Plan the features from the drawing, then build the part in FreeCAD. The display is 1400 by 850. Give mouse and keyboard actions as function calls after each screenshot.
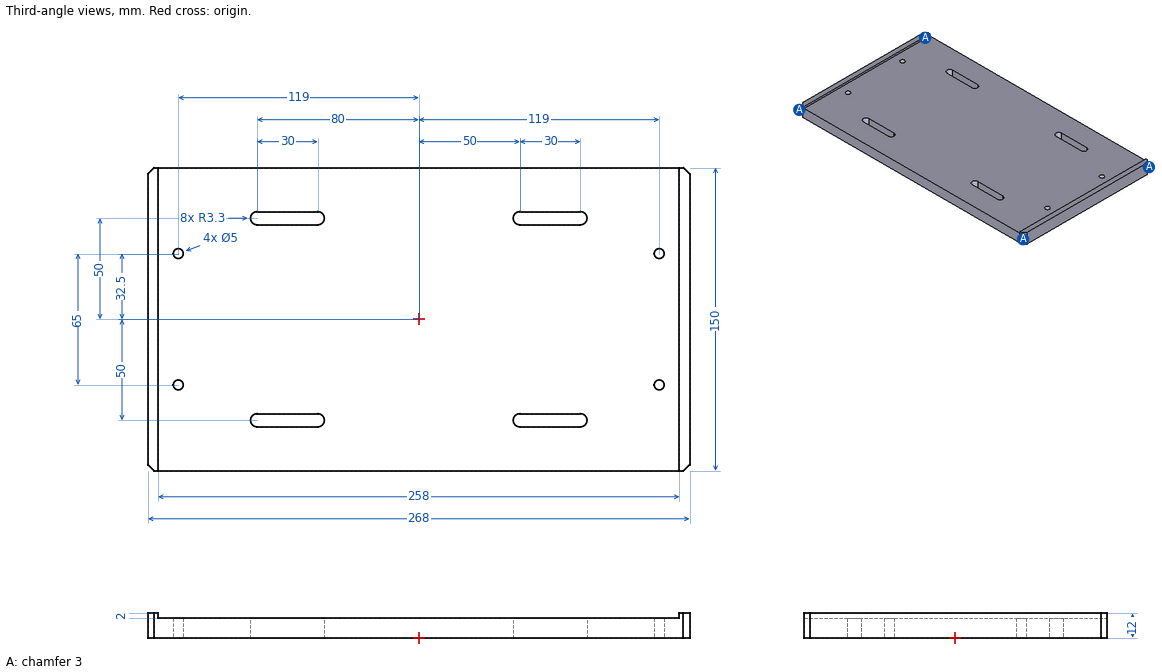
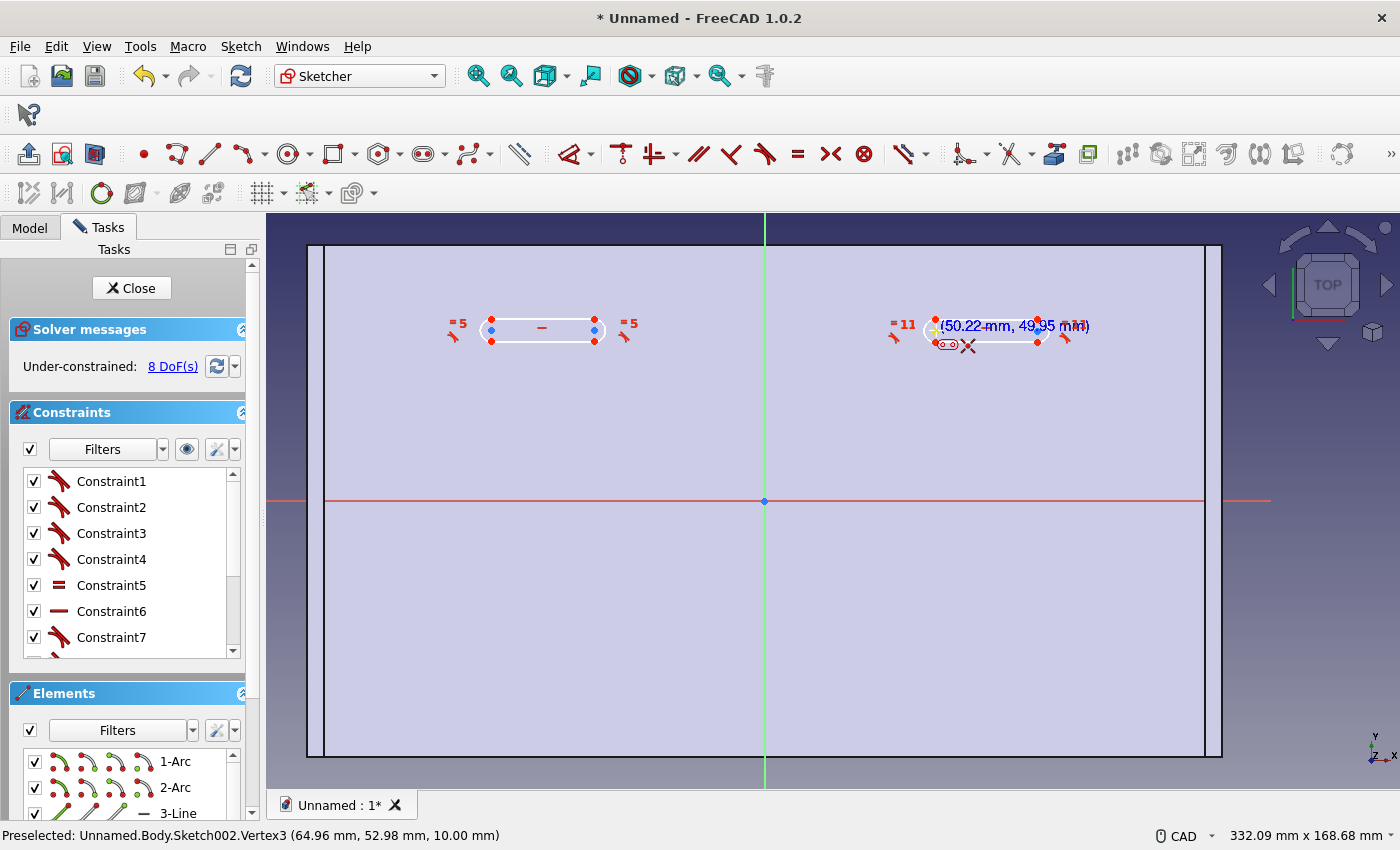
scroll(492, 672, up, 4)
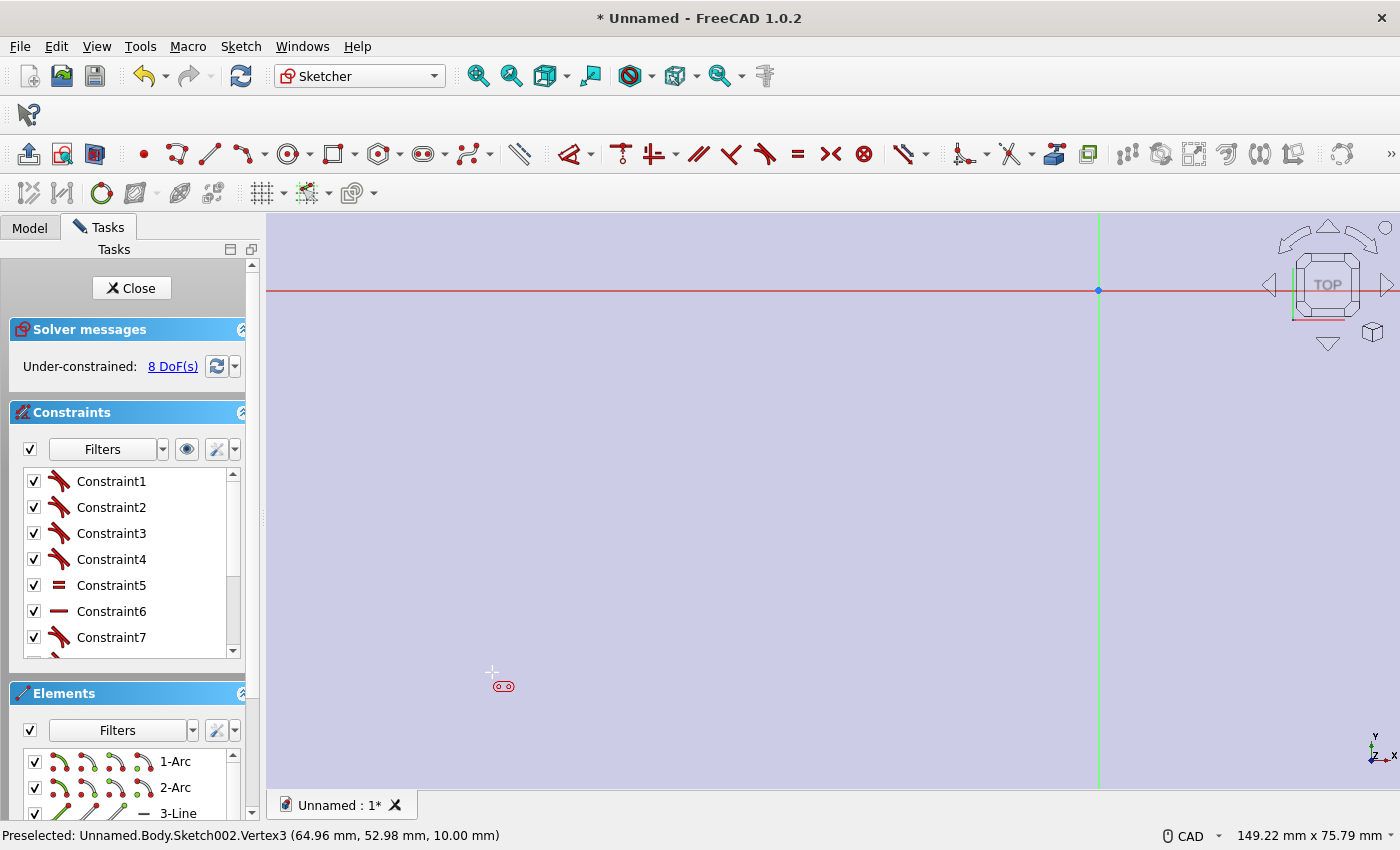
click(491, 671)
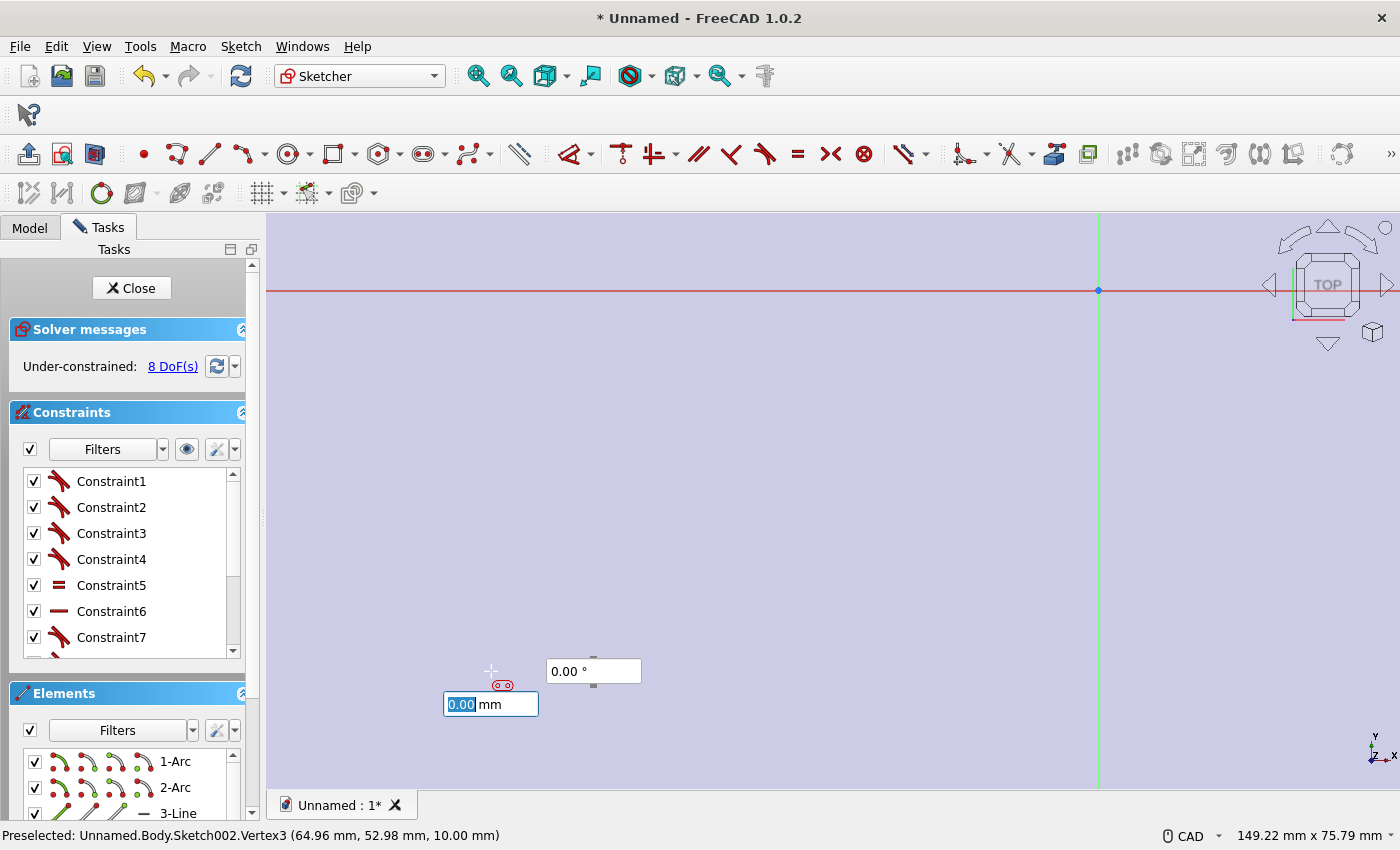
click(719, 671)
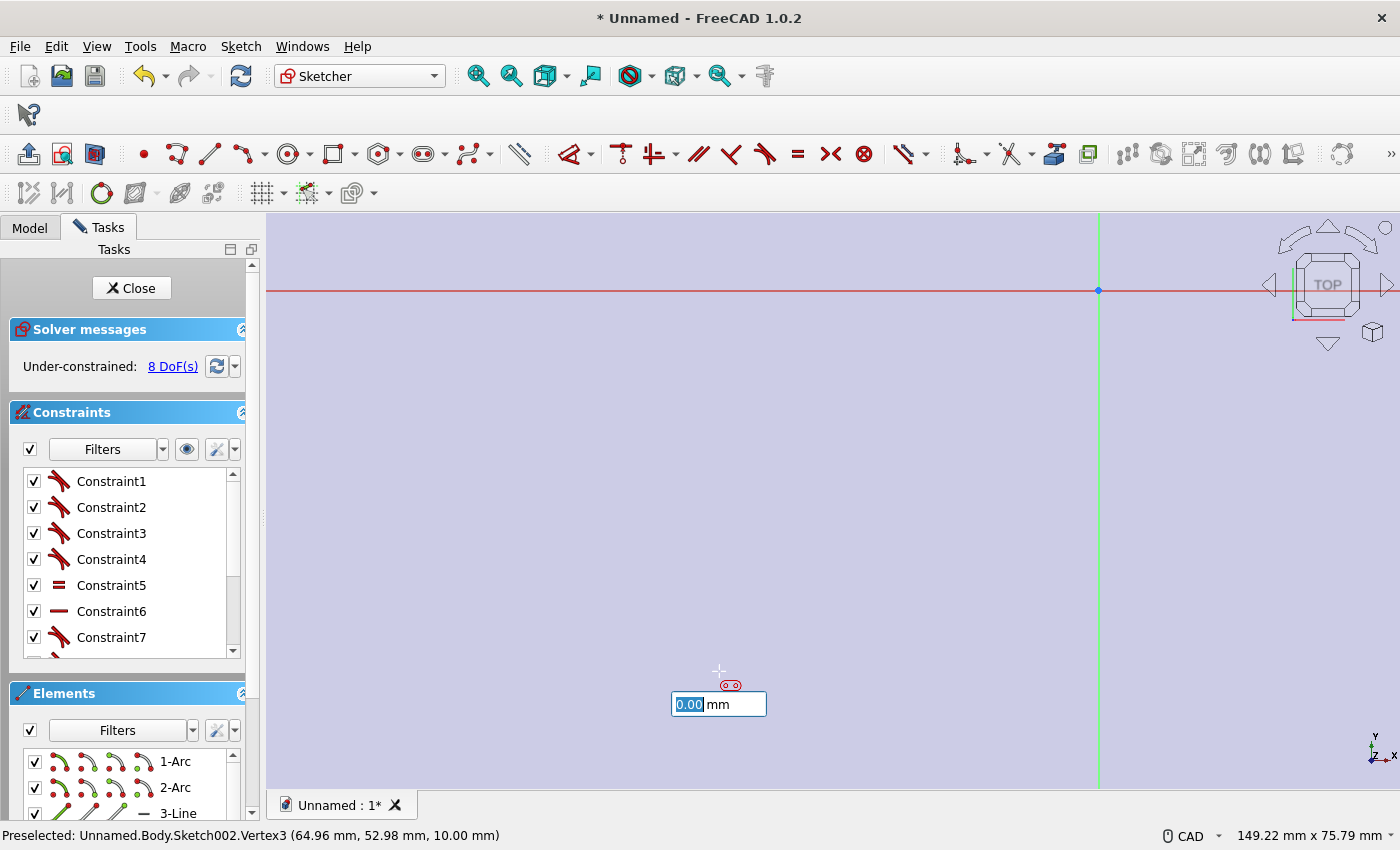
click(605, 646)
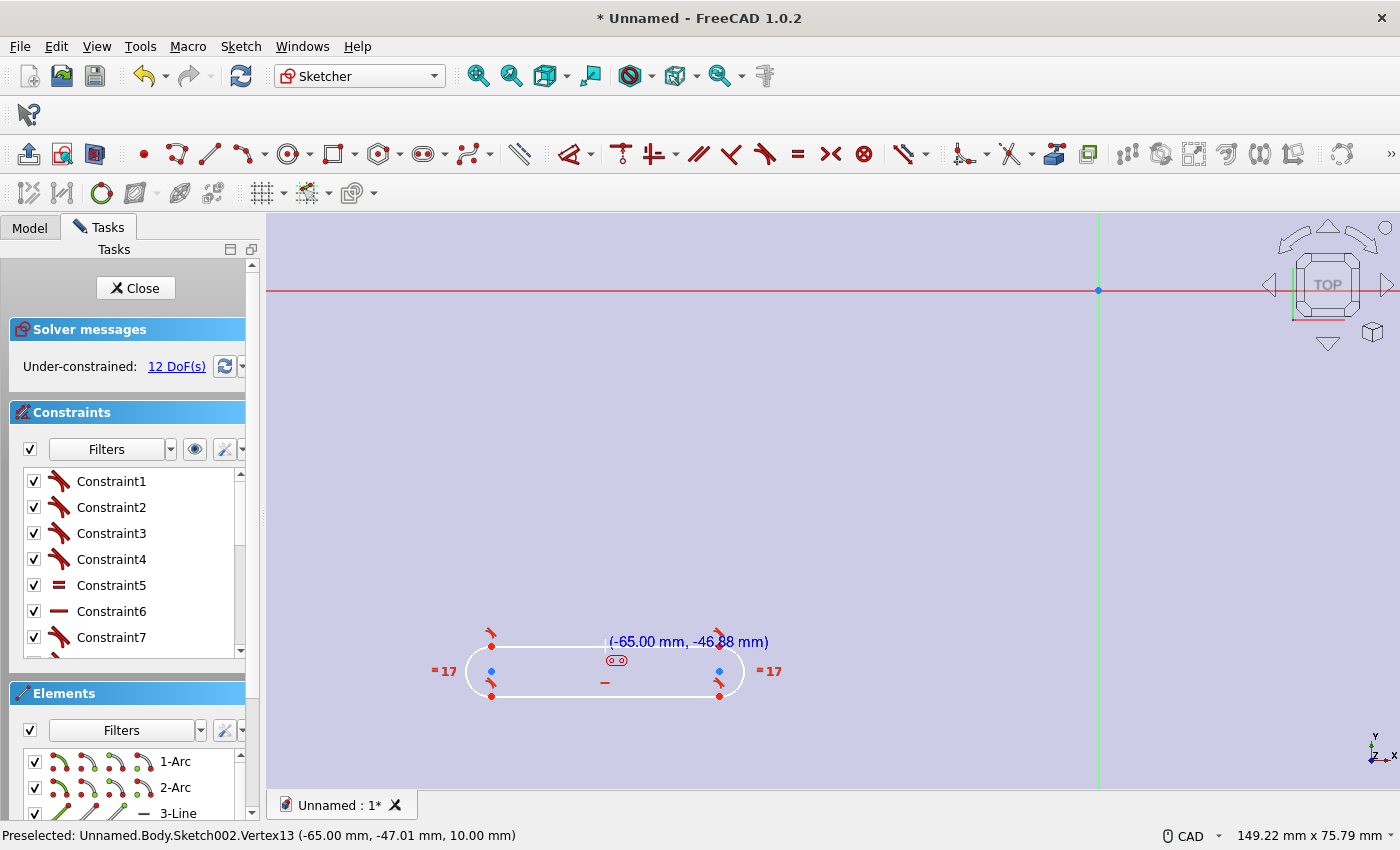
scroll(492, 673, down, 4)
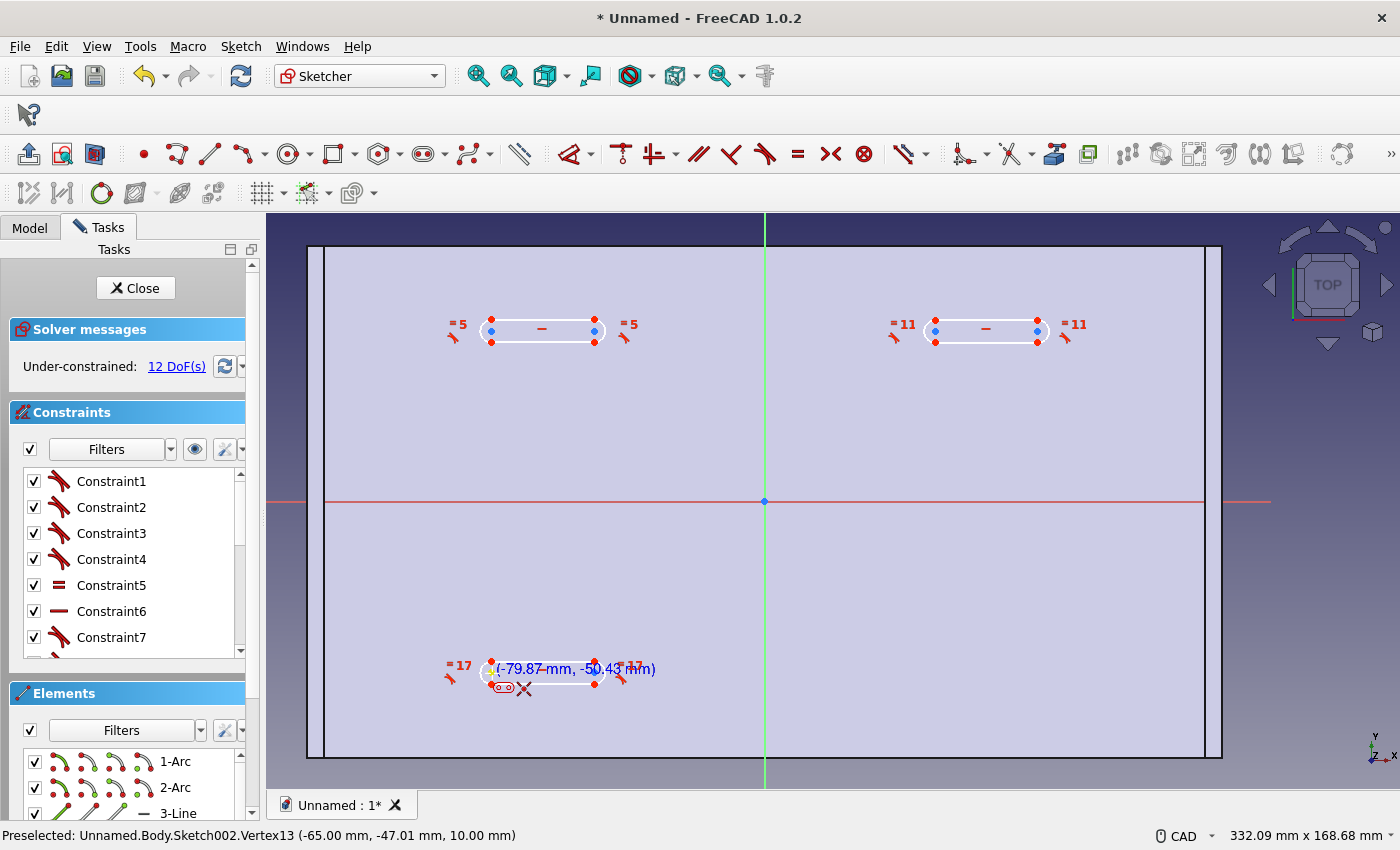
scroll(936, 672, up, 4)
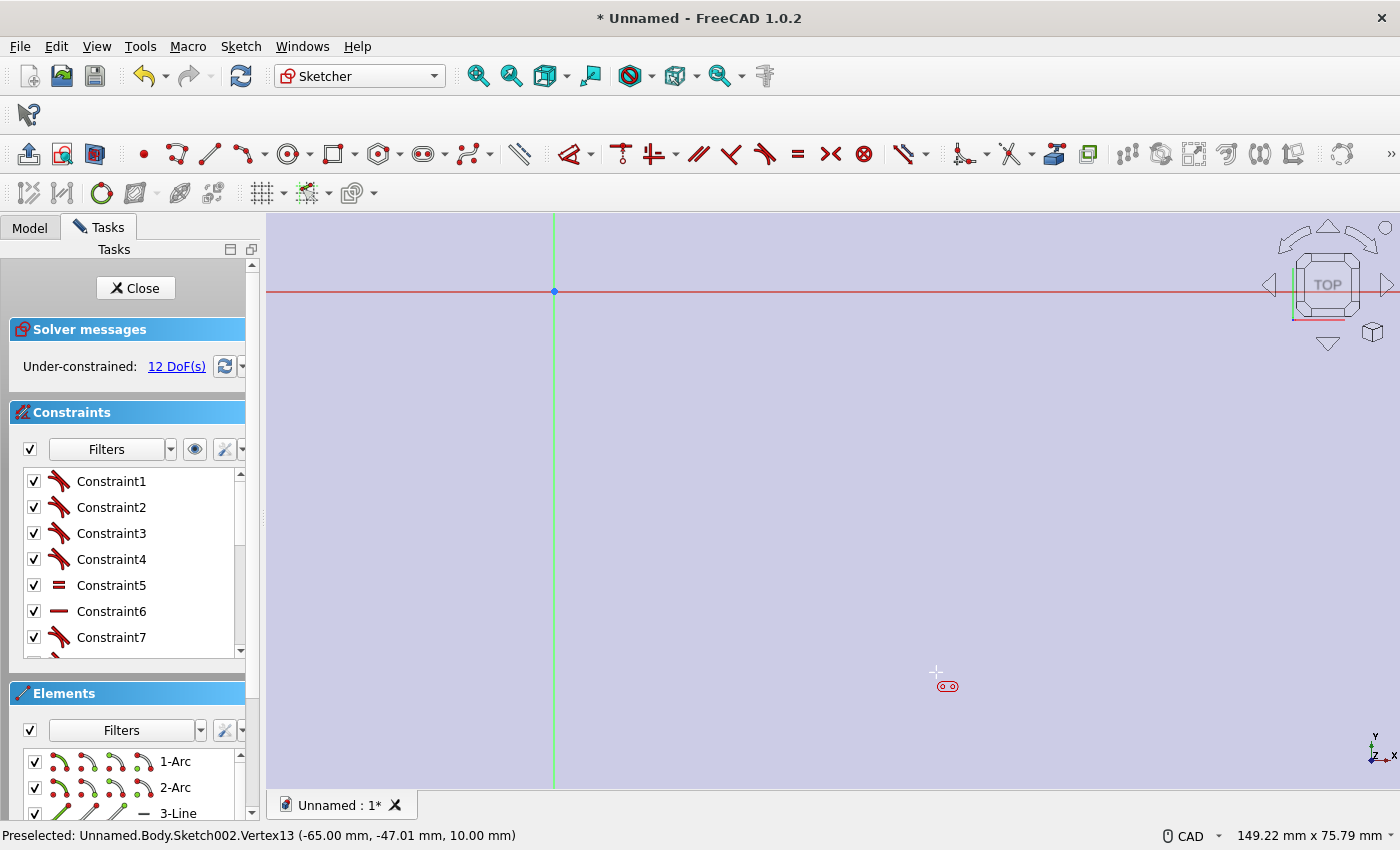
click(934, 672)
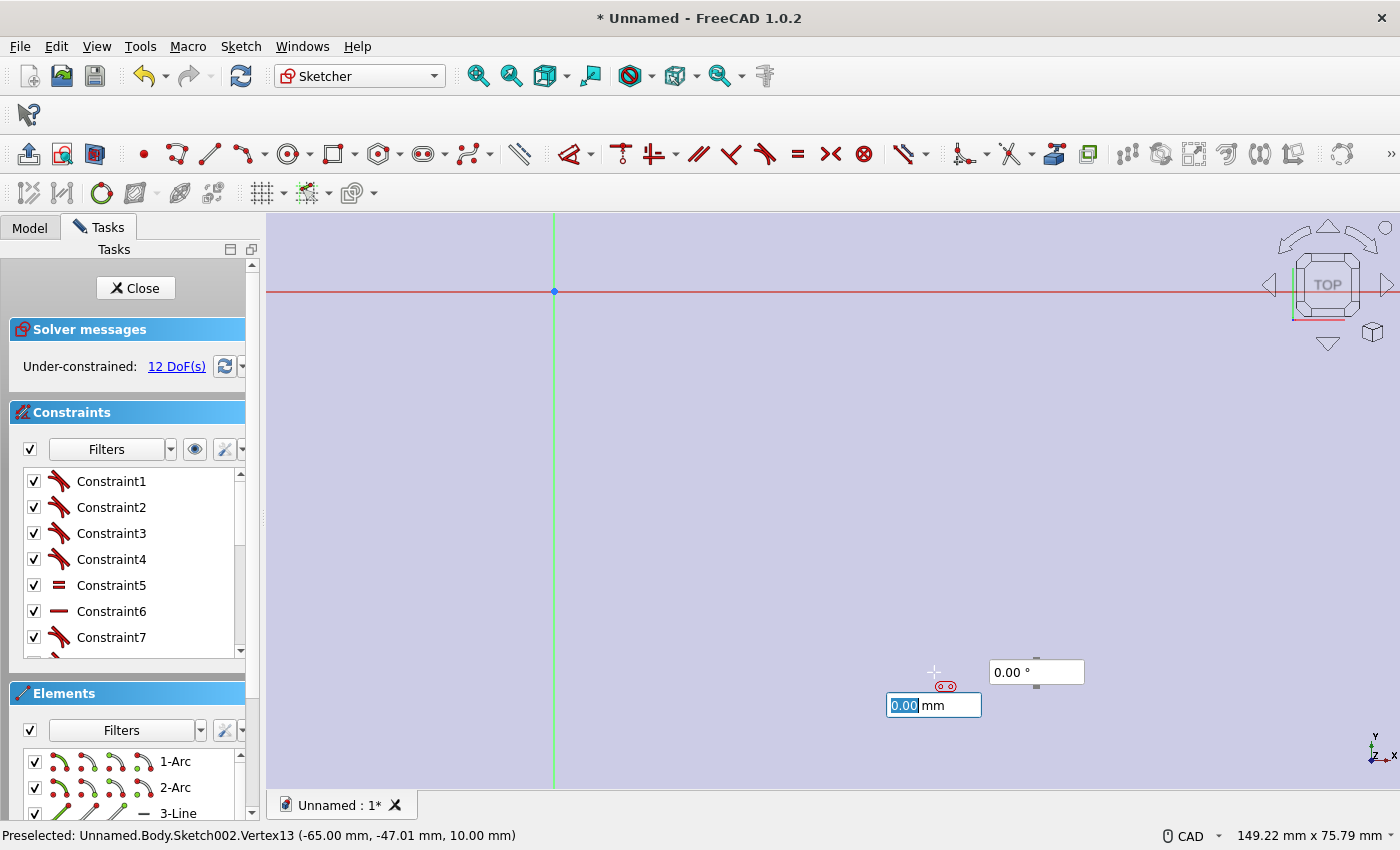
click(1162, 672)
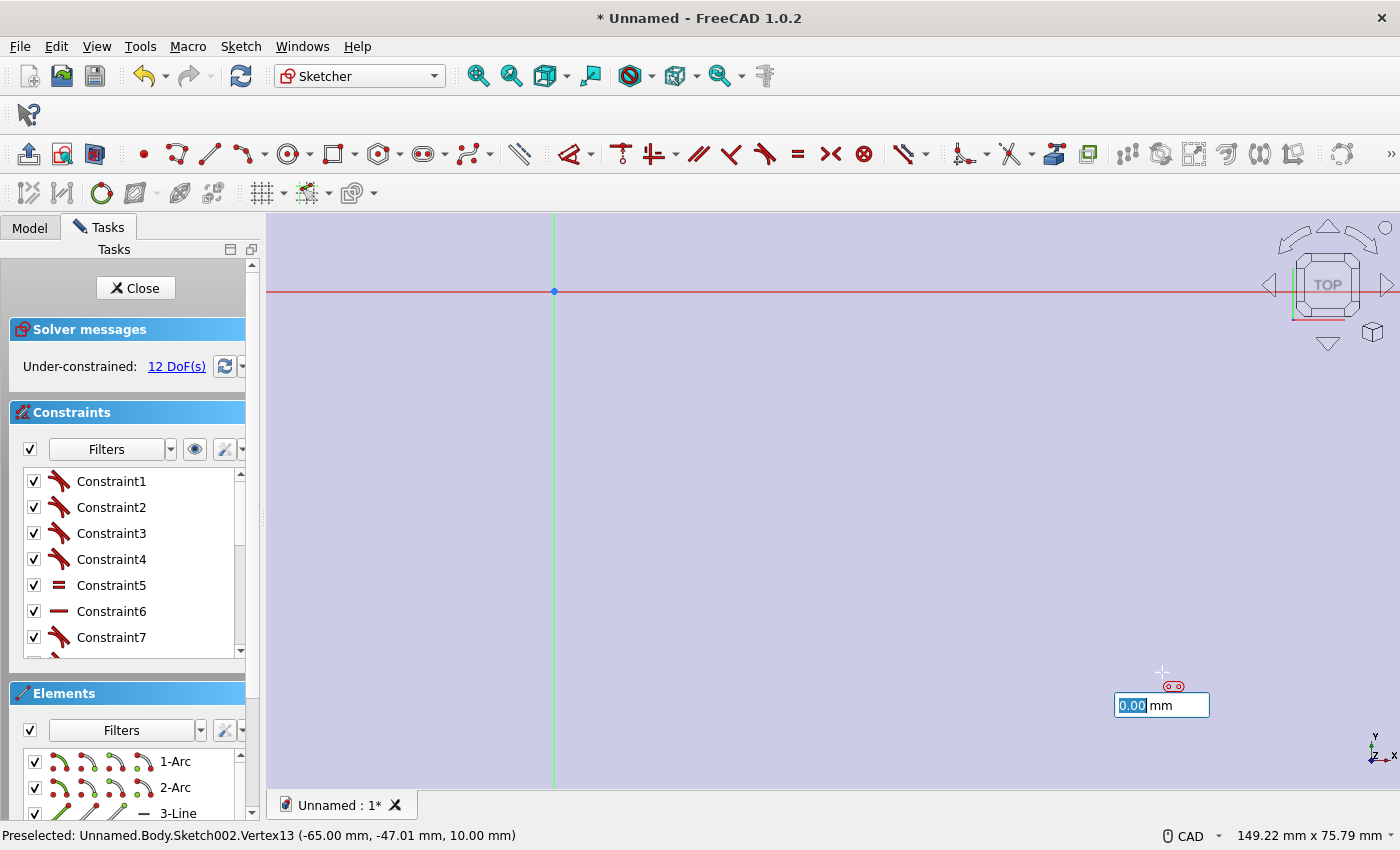
click(1048, 647)
key(Escape)